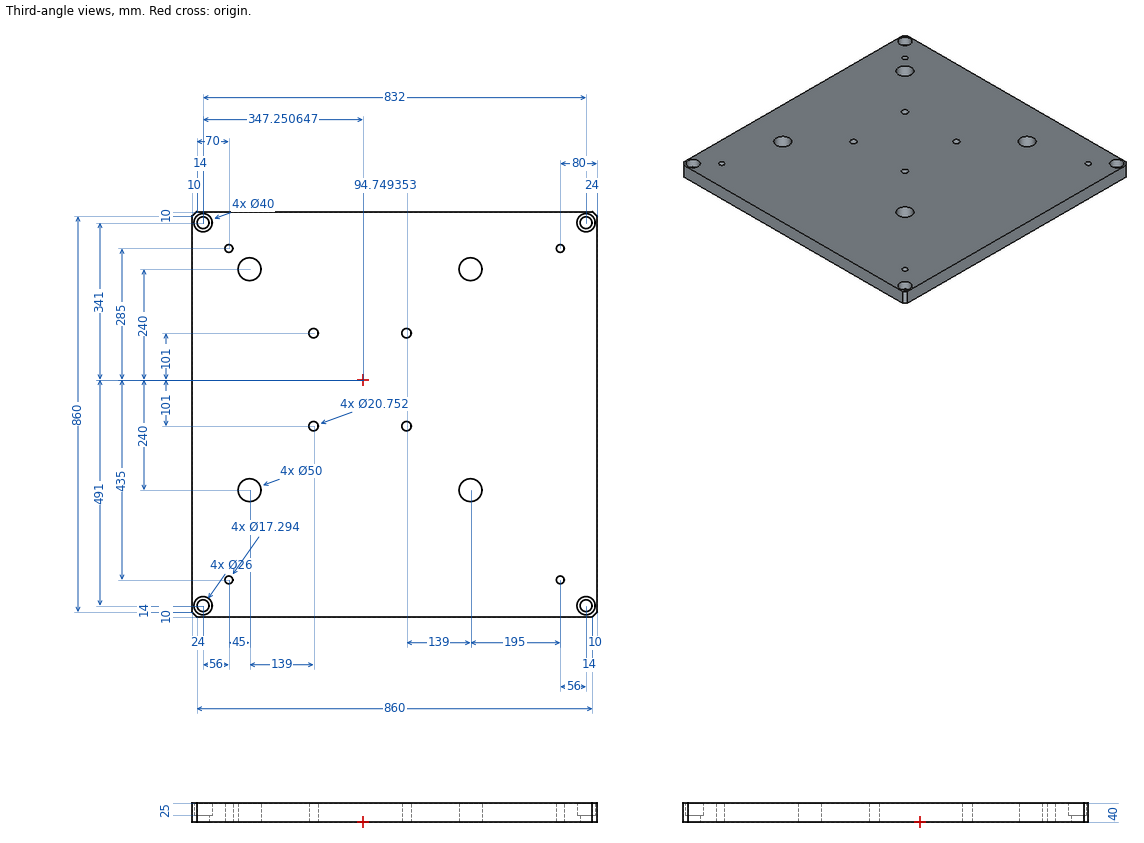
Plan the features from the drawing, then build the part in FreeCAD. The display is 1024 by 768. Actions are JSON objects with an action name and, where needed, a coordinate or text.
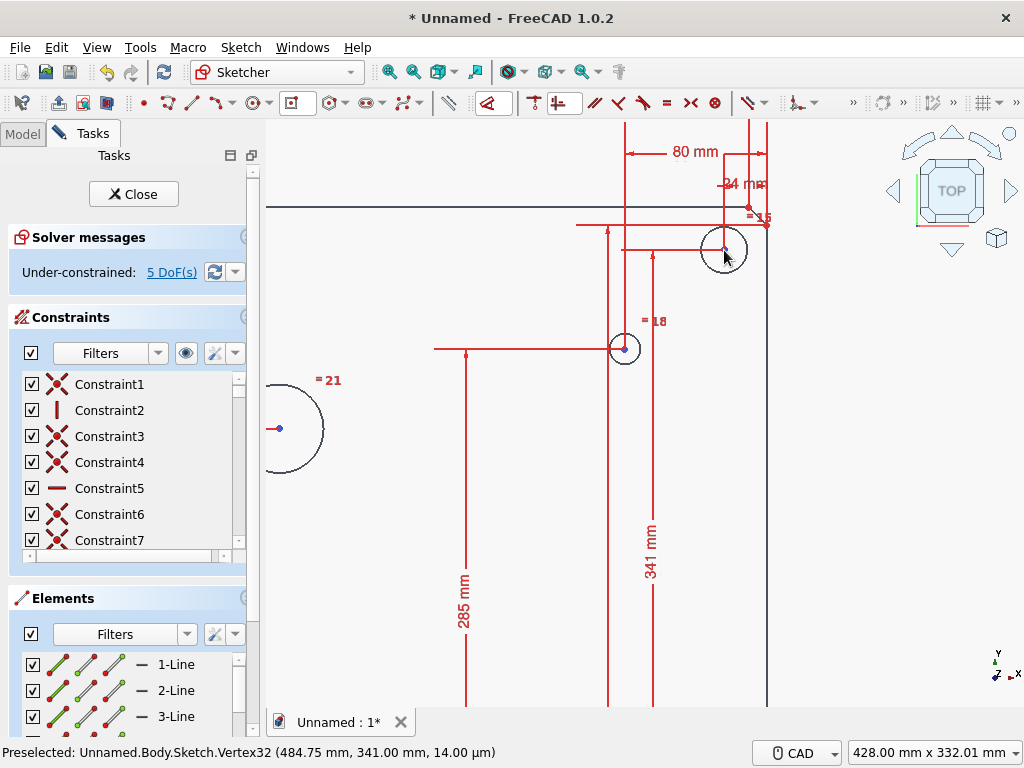
{"action": "scroll", "coordinate": [769, 225], "scroll_direction": "down", "scroll_amount": 7}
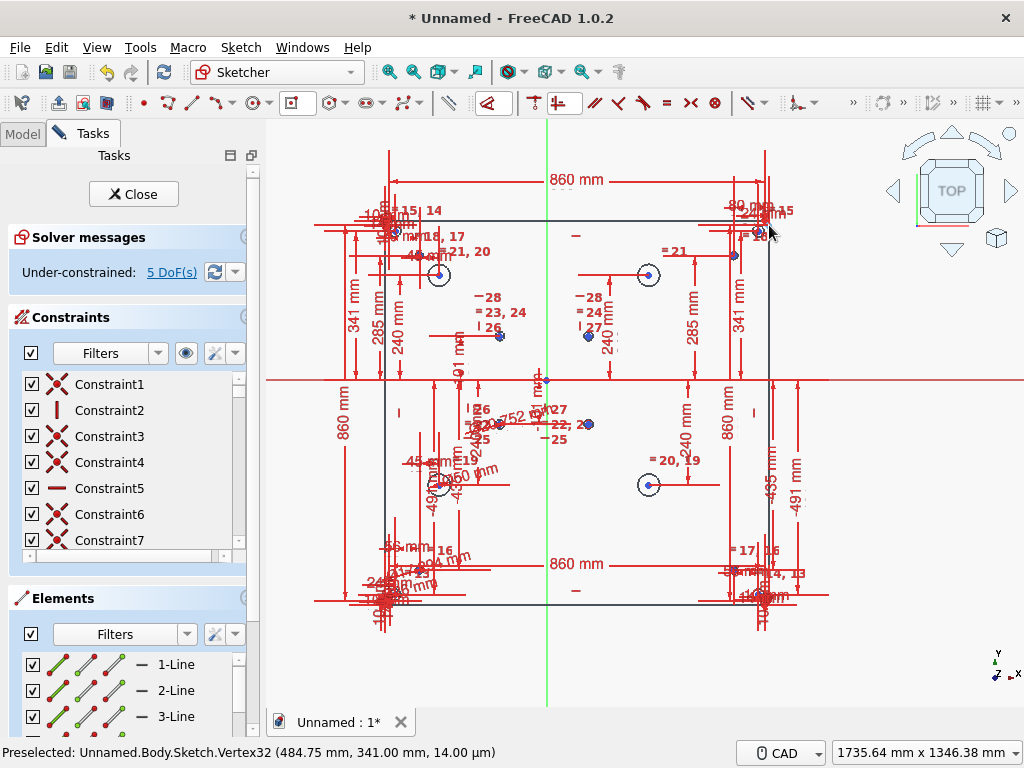
{"action": "left_click", "coordinate": [439, 485]}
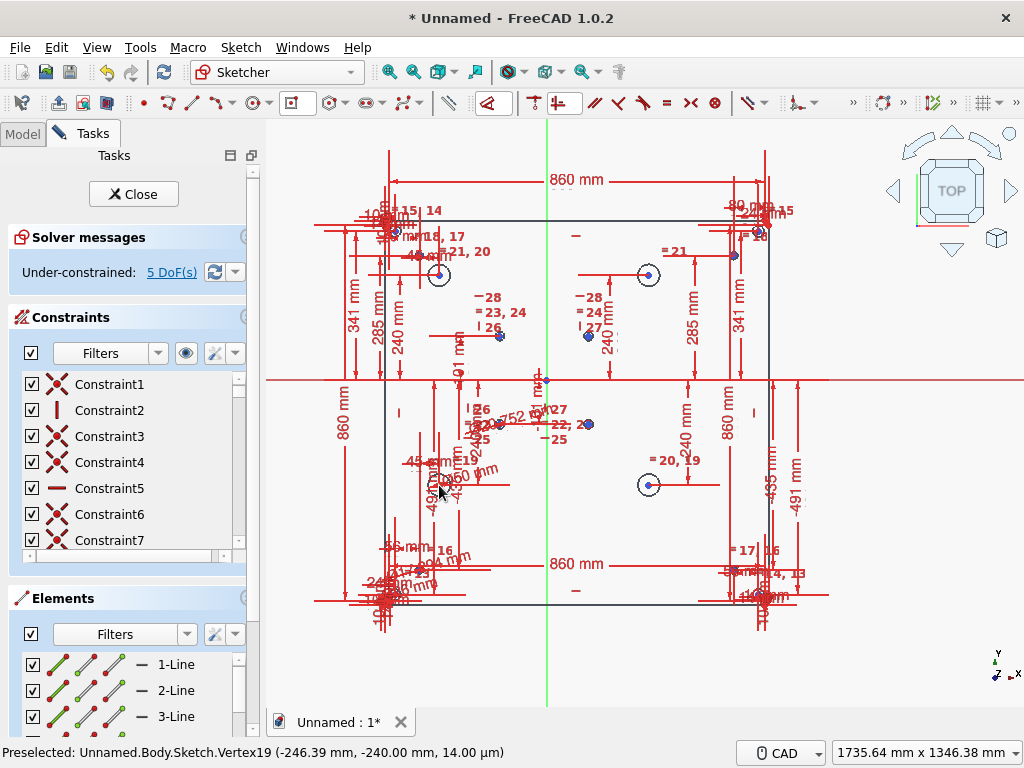
{"action": "left_click", "coordinate": [500, 424]}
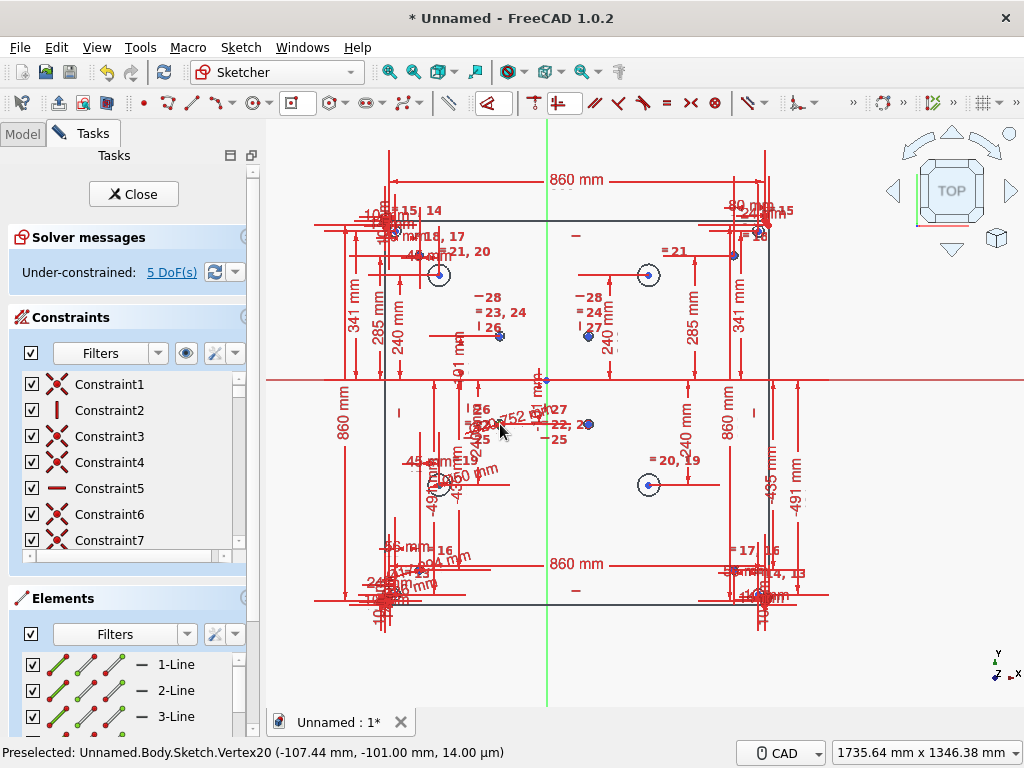
{"action": "key", "text": "l"}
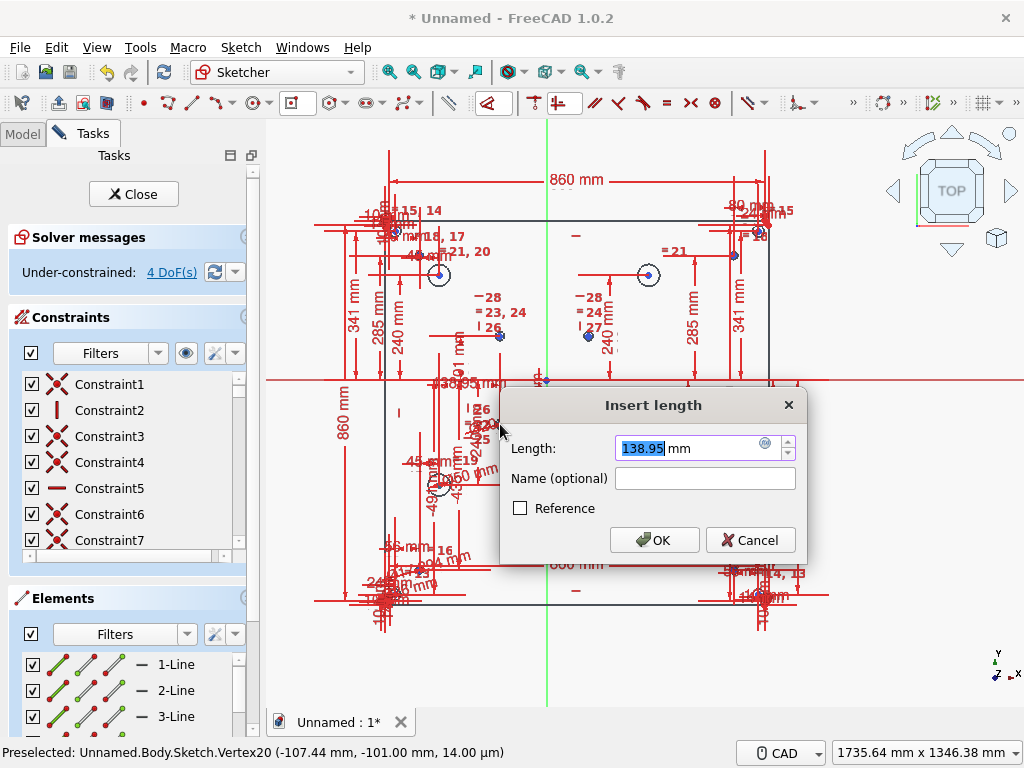
{"action": "type", "text": "139"}
{"action": "key", "text": "Return"}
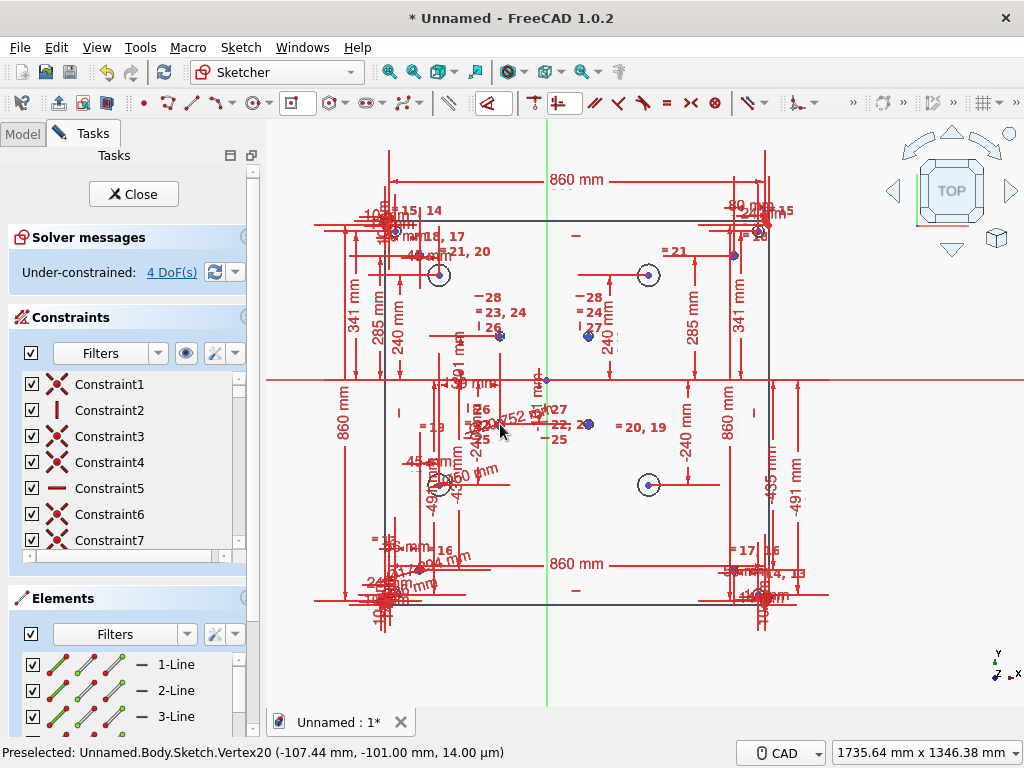
{"action": "left_click", "coordinate": [734, 570]}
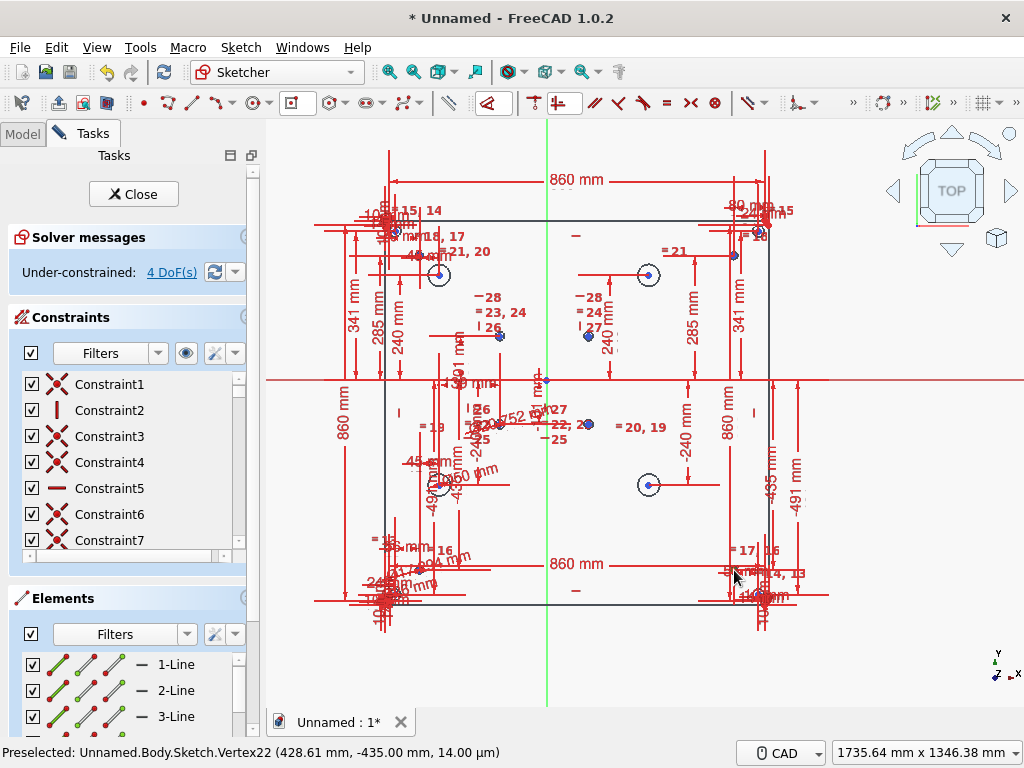
{"action": "left_click", "coordinate": [649, 485]}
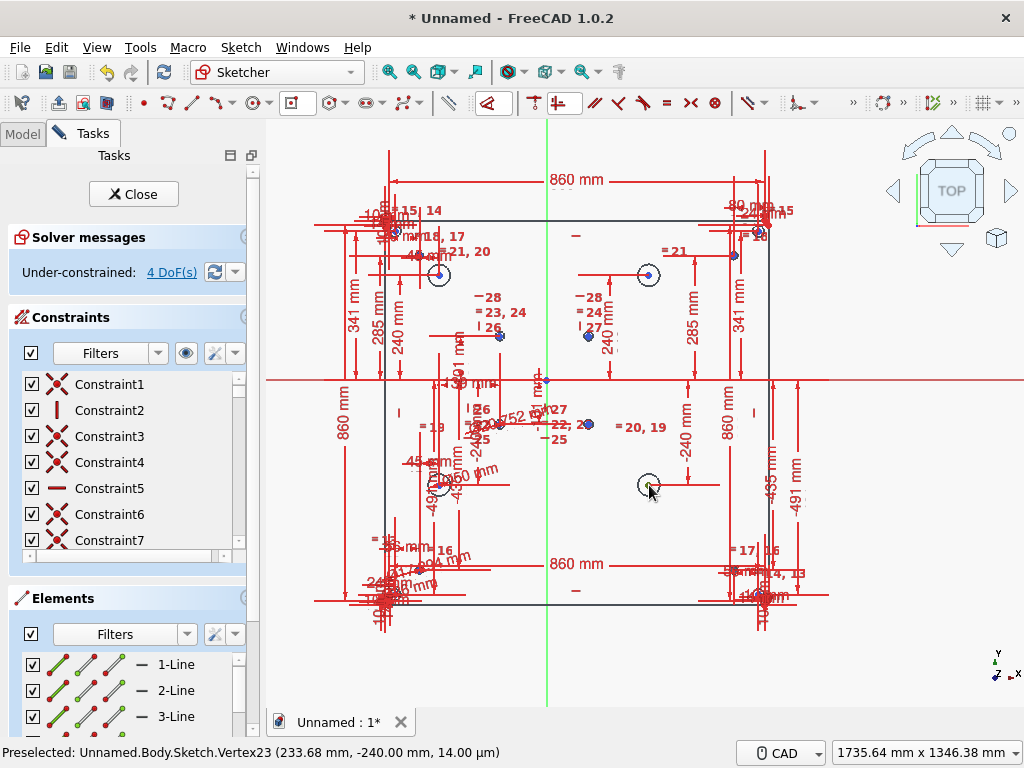
{"action": "key", "text": "l"}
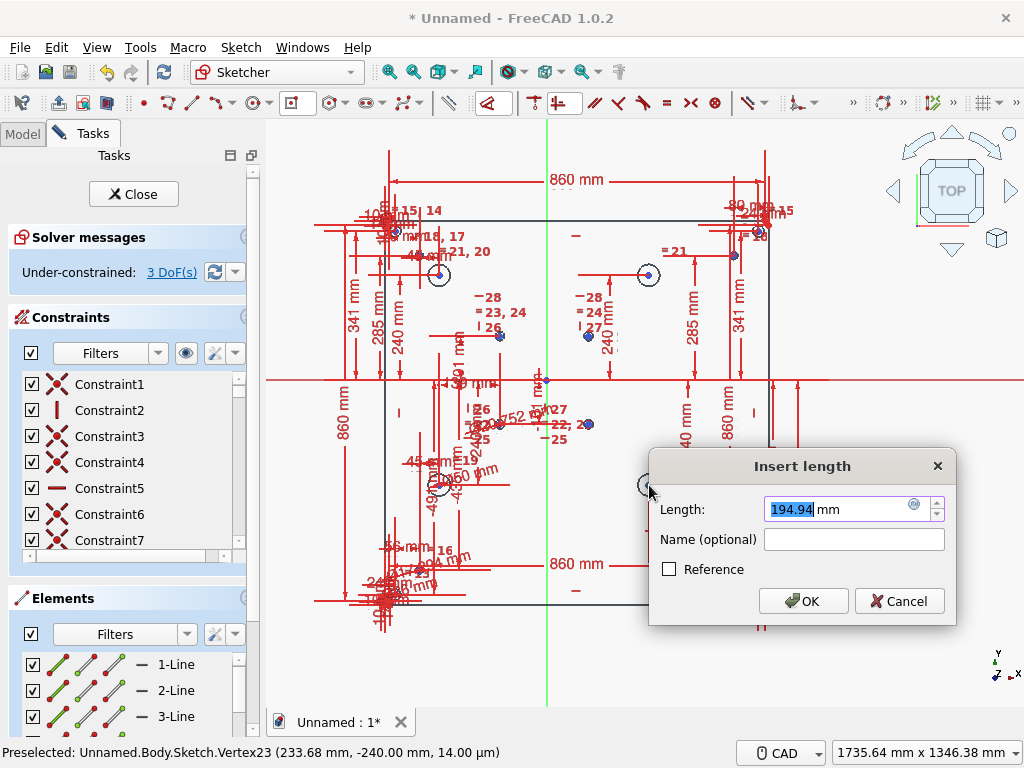
{"action": "type", "text": "195"}
{"action": "key", "text": "Return"}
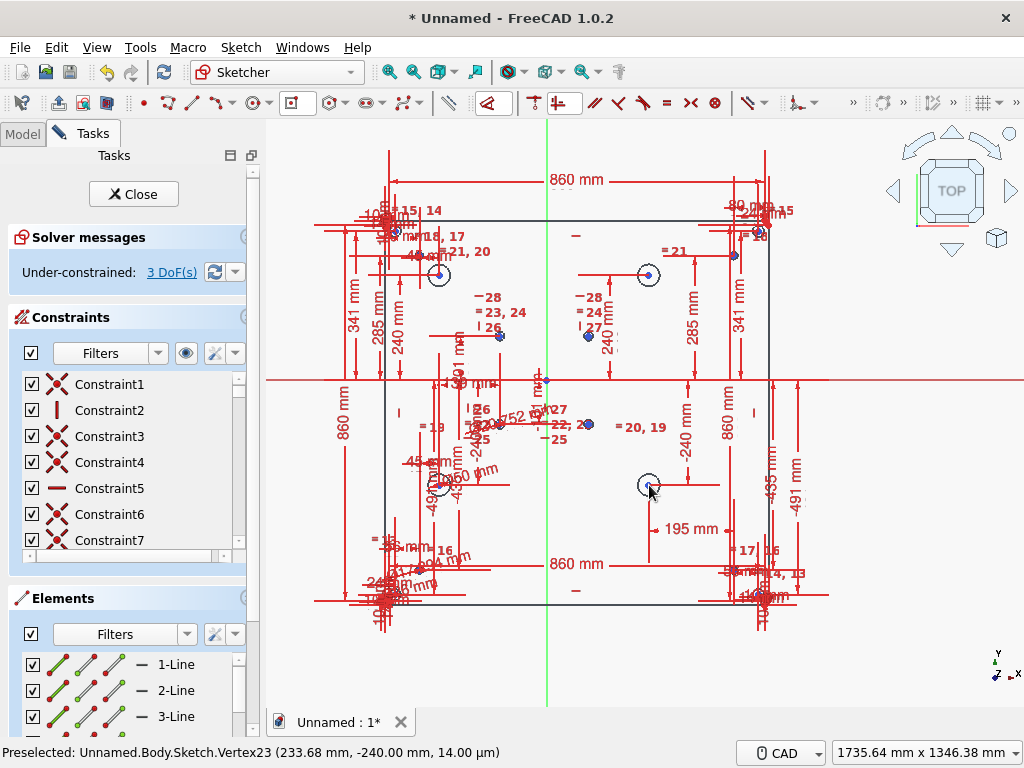
{"action": "left_click", "coordinate": [649, 485]}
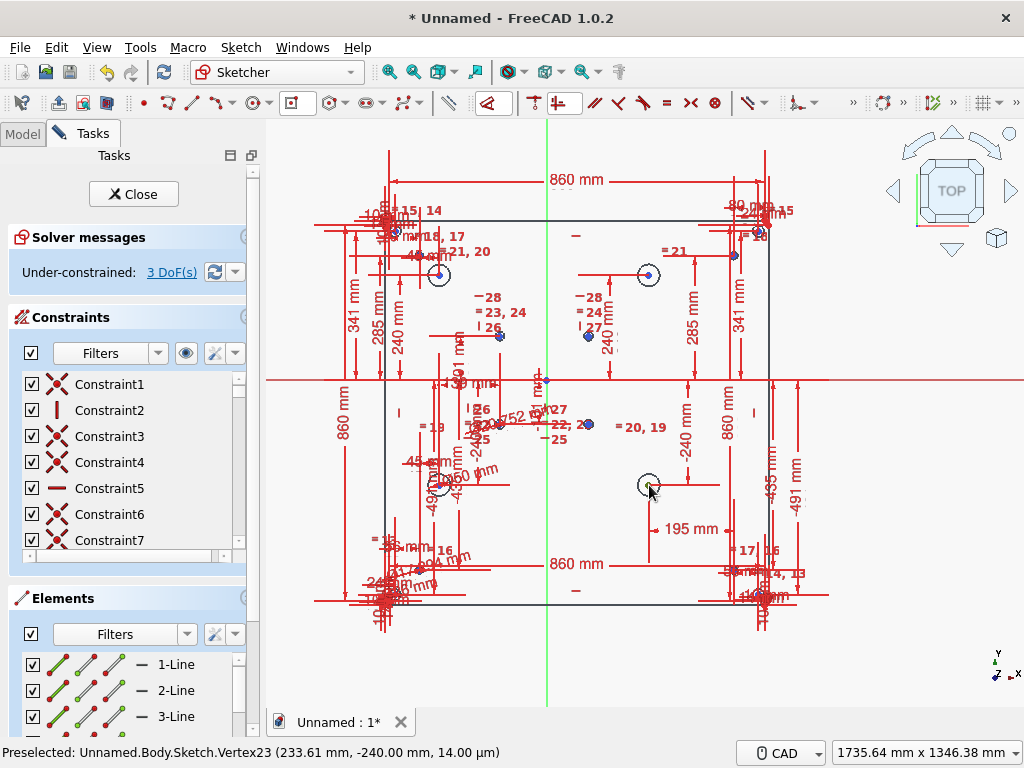
{"action": "left_click", "coordinate": [589, 424]}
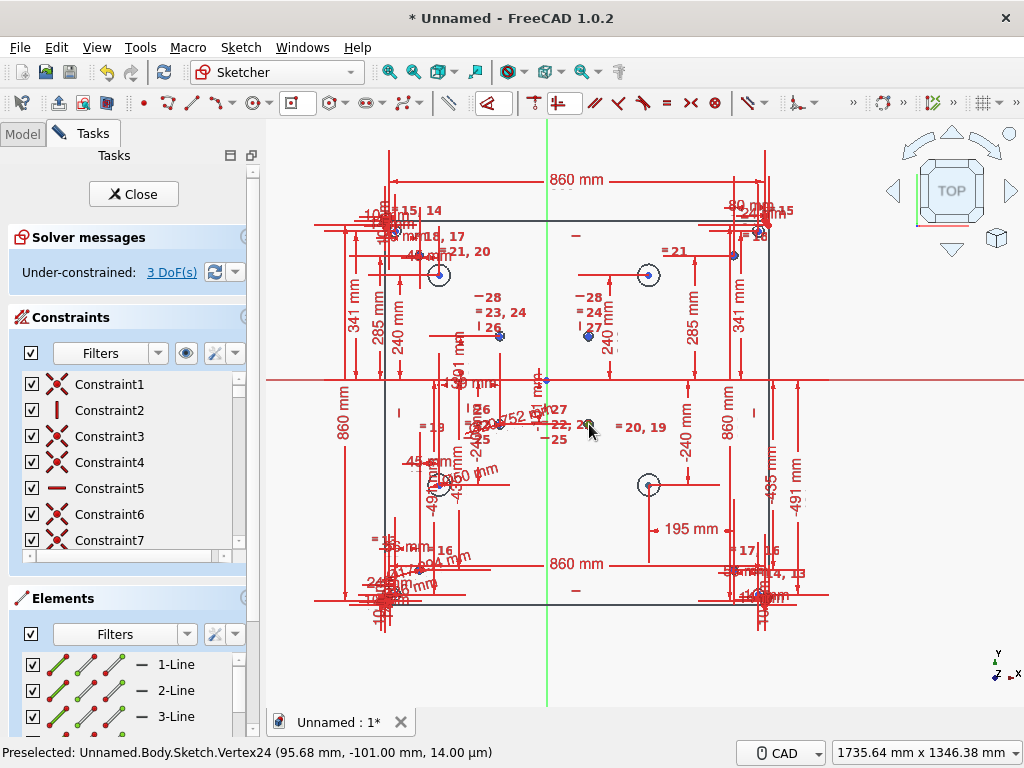
{"action": "key", "text": "l"}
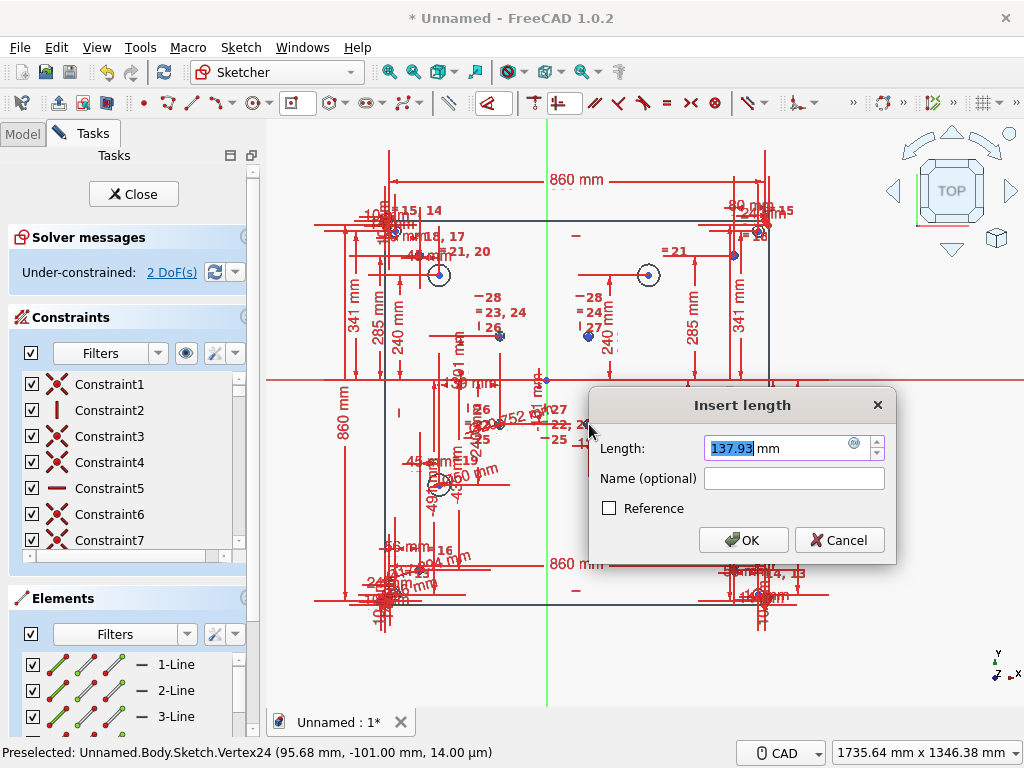
{"action": "type", "text": "139"}
{"action": "key", "text": "Return"}